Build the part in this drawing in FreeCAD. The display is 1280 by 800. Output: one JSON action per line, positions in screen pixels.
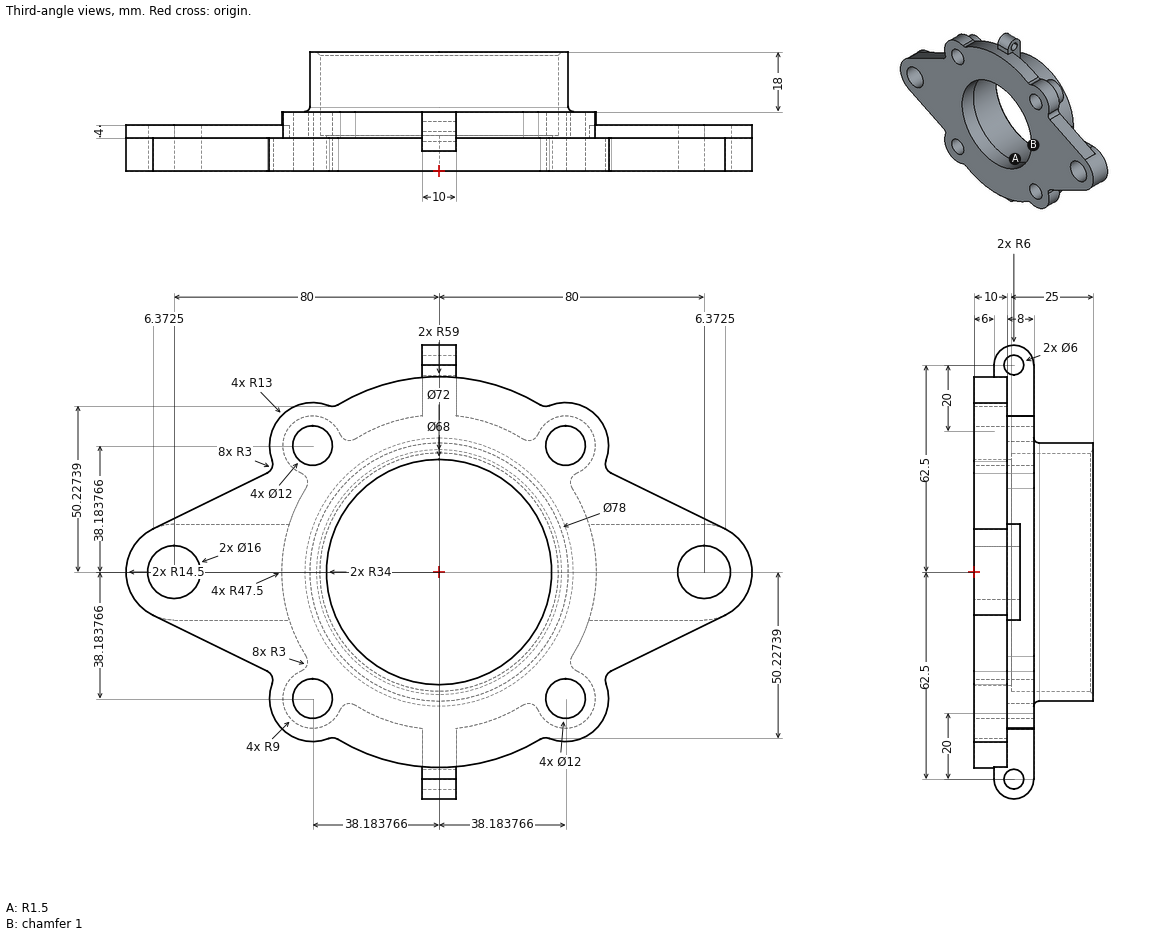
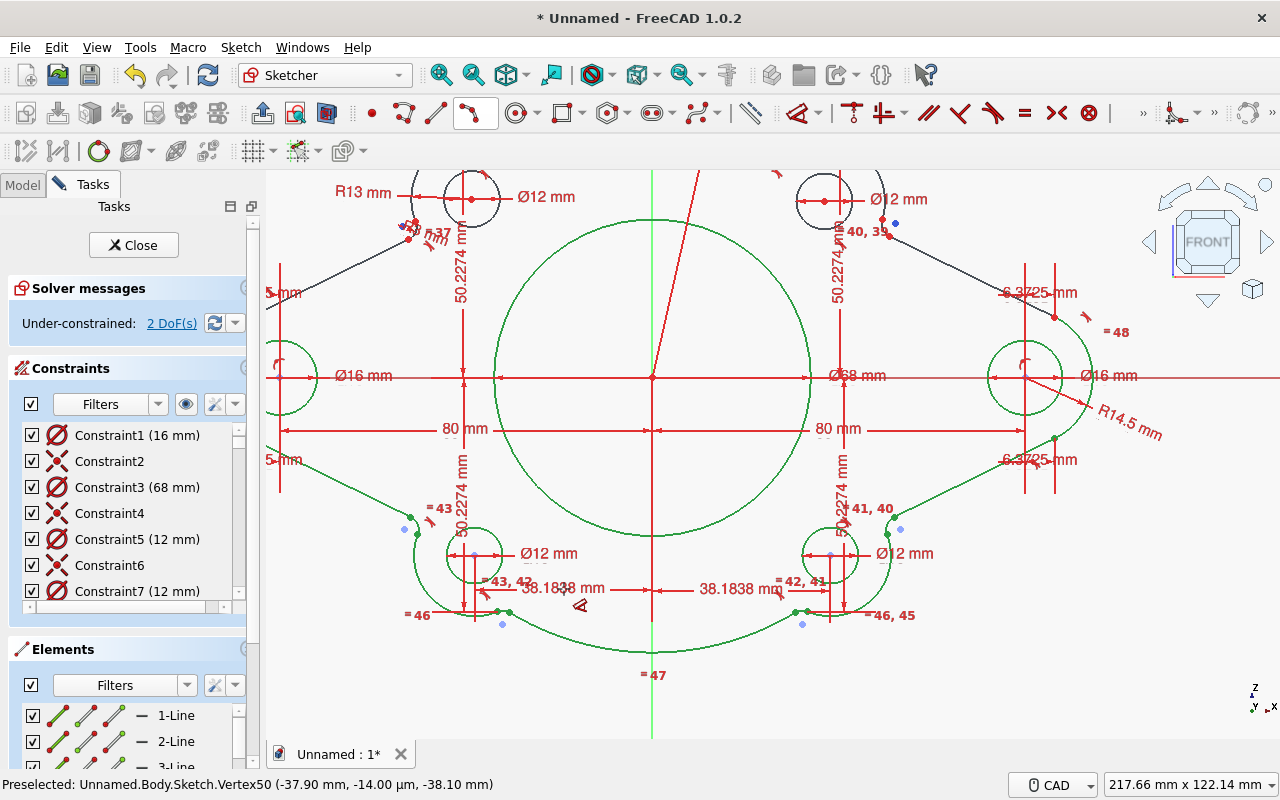
{"action": "left_click", "coordinate": [824, 201]}
{"action": "left_click", "coordinate": [738, 412]}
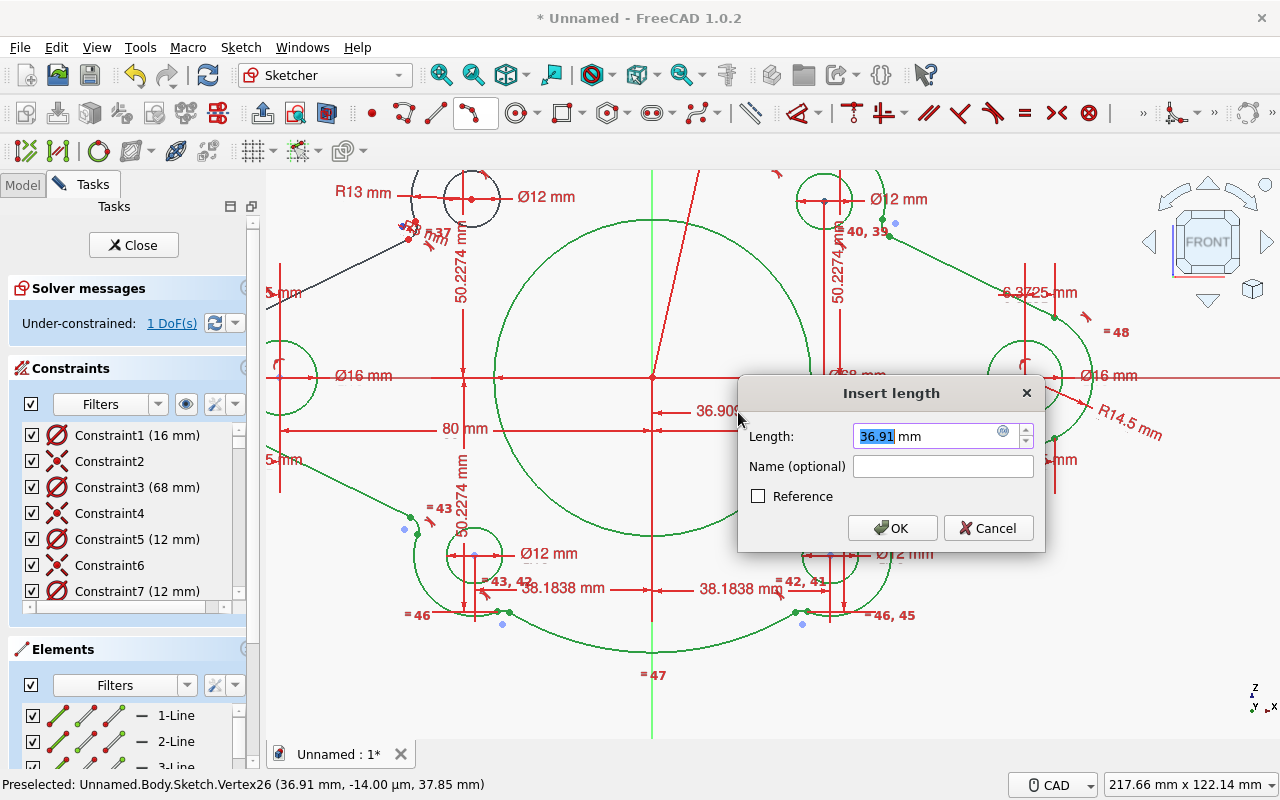
{"action": "type", "text": "38.183766"}
{"action": "key", "text": "Return"}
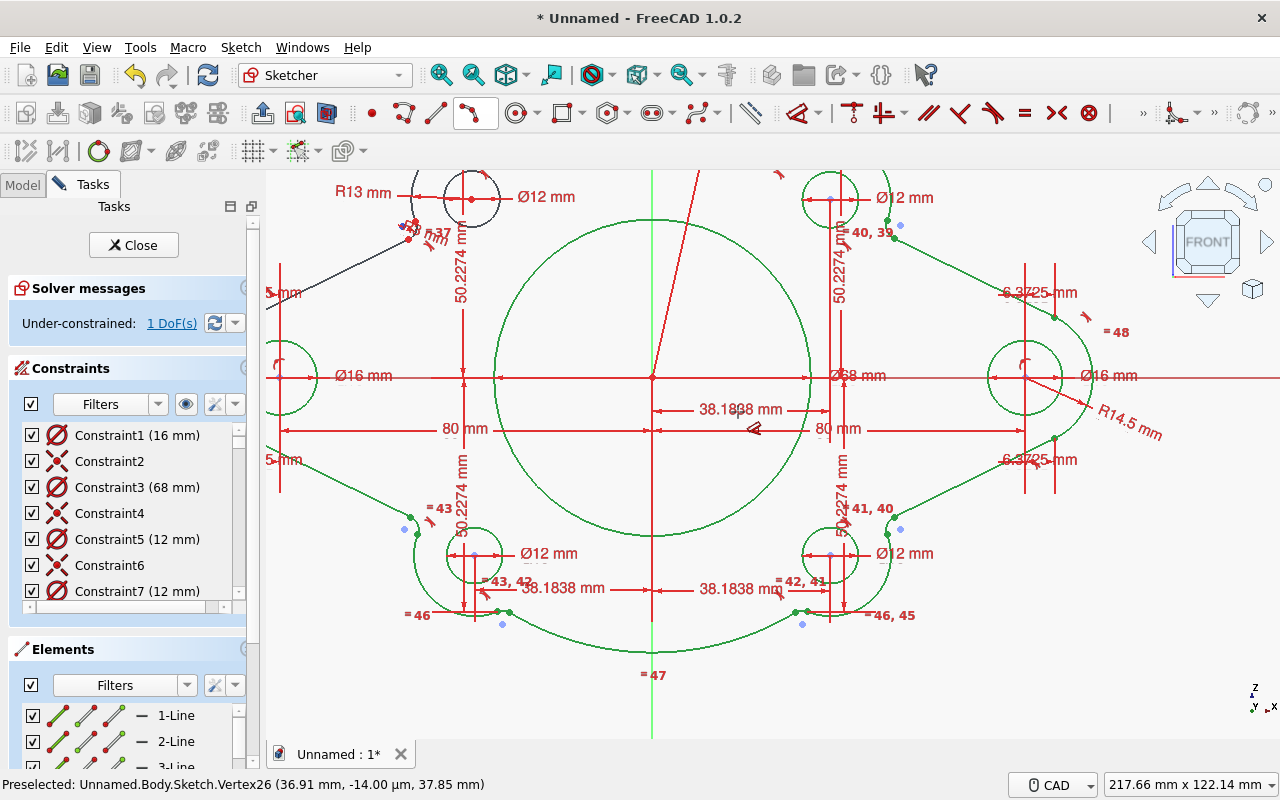
{"action": "left_click", "coordinate": [472, 199]}
{"action": "left_click", "coordinate": [562, 412]}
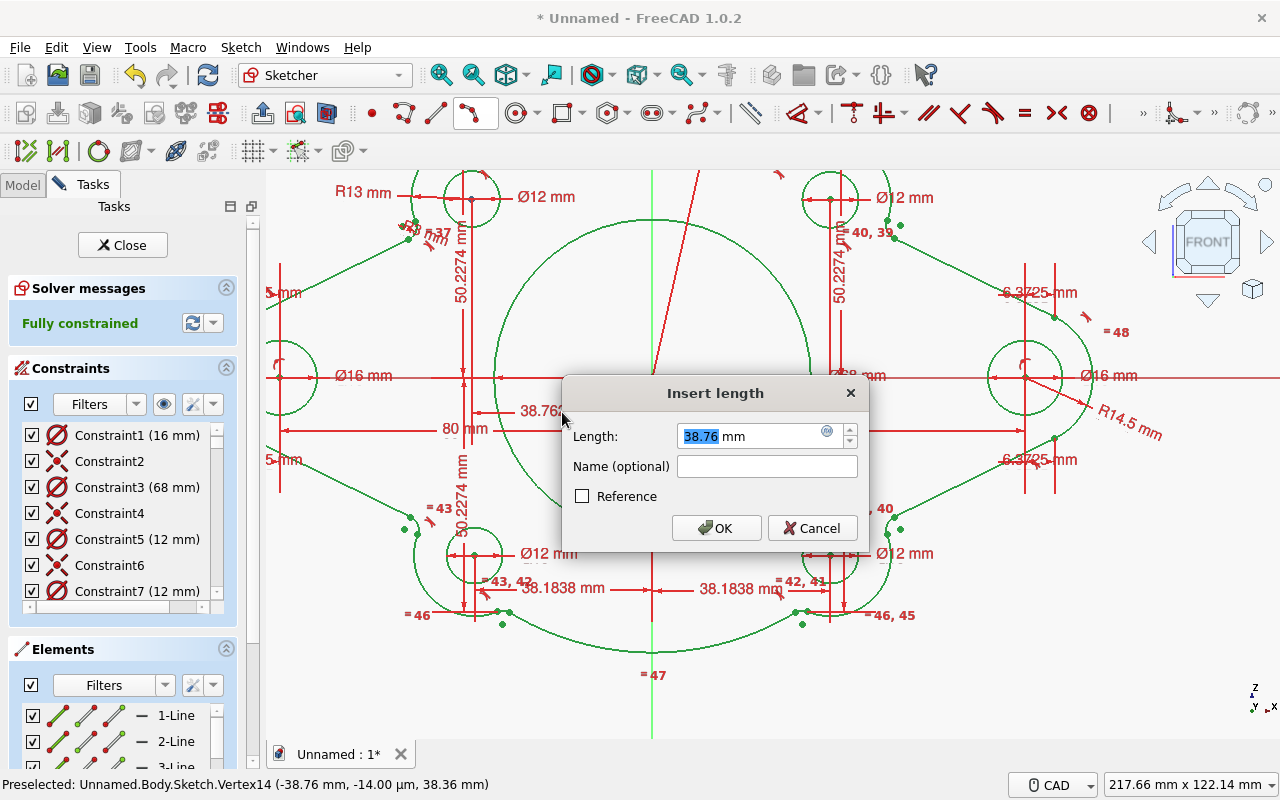
{"action": "type", "text": "38.183766"}
{"action": "key", "text": "Return"}
{"action": "key", "text": "Escape"}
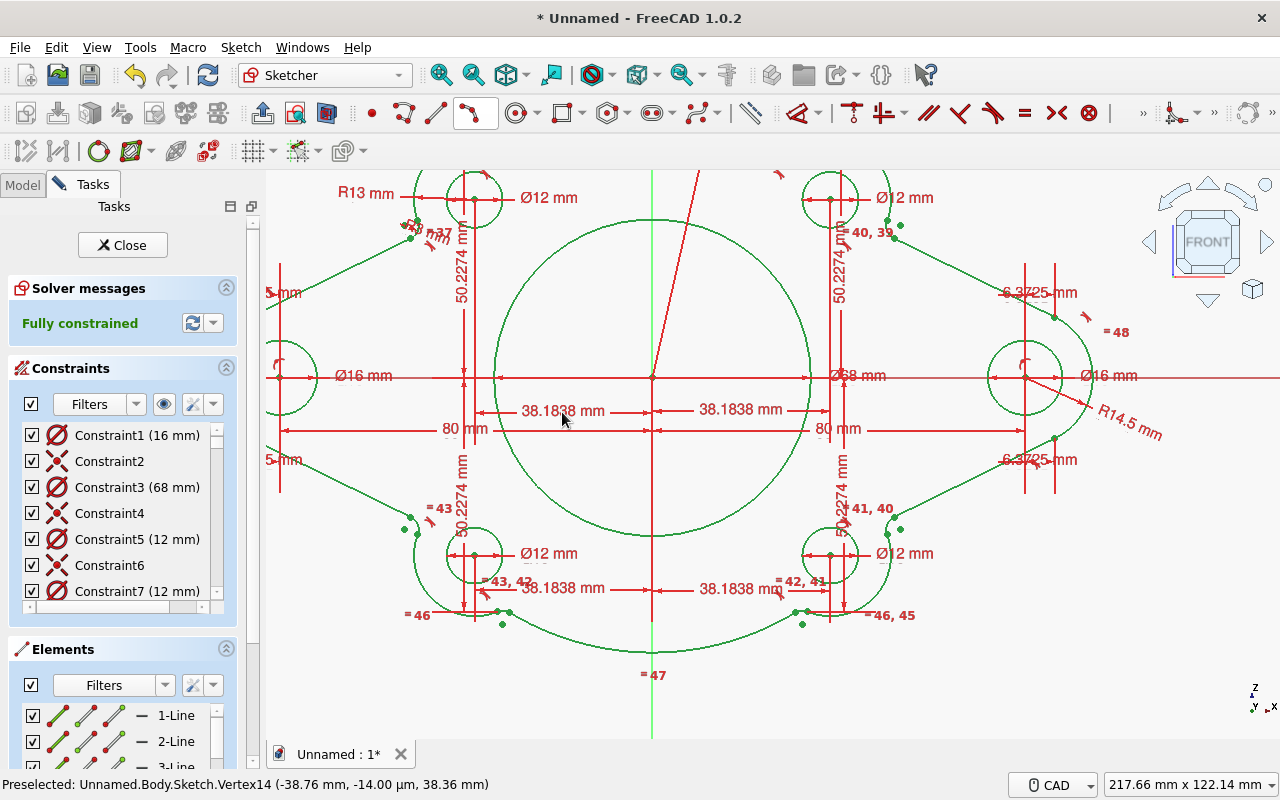
{"action": "left_click", "coordinate": [123, 245]}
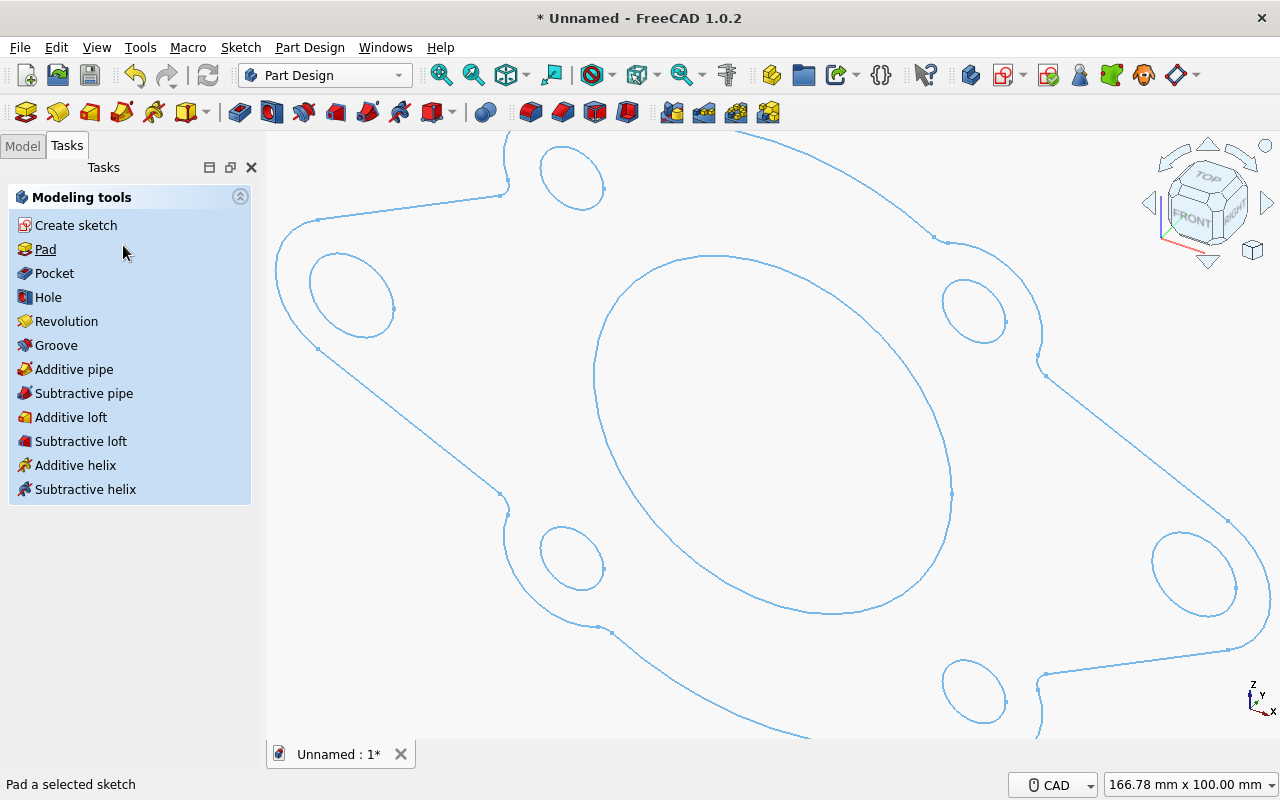
{"action": "left_click", "coordinate": [26, 112]}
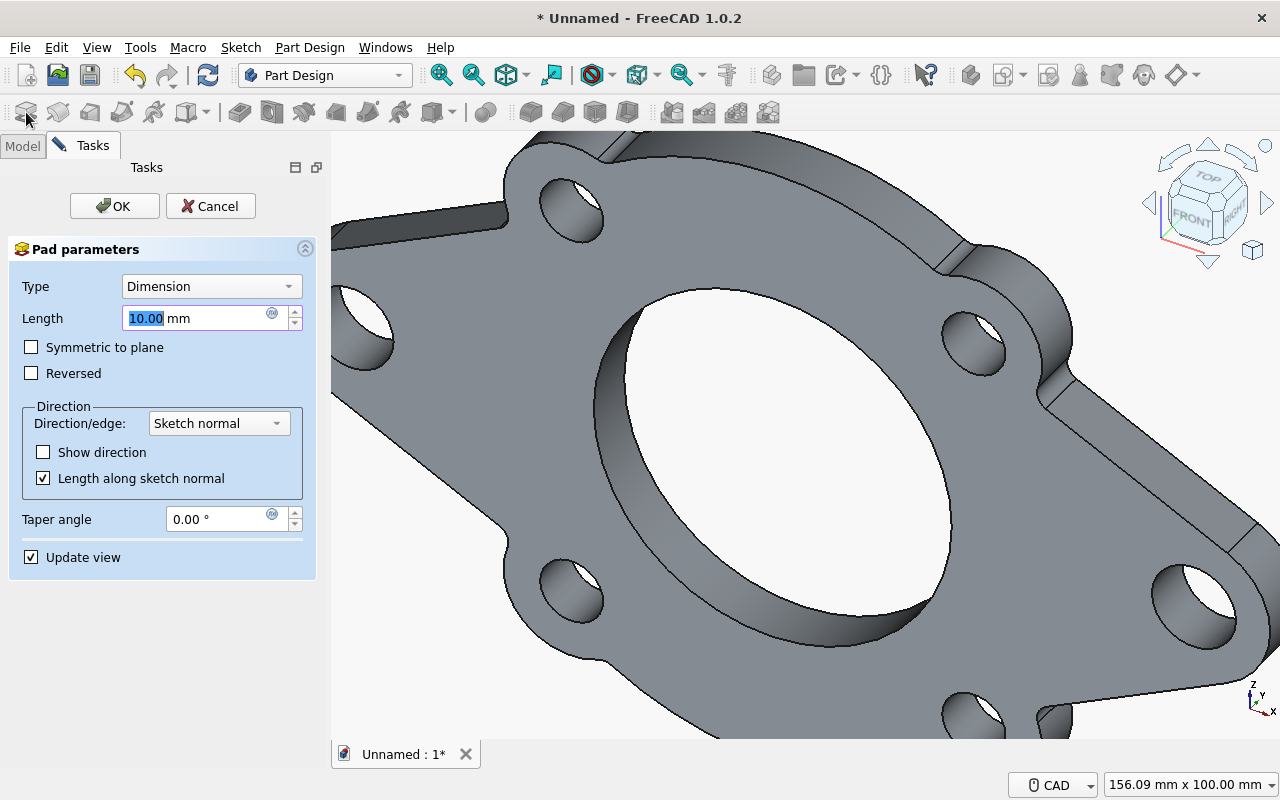
{"action": "type", "text": "10"}
{"action": "key", "text": "Tab"}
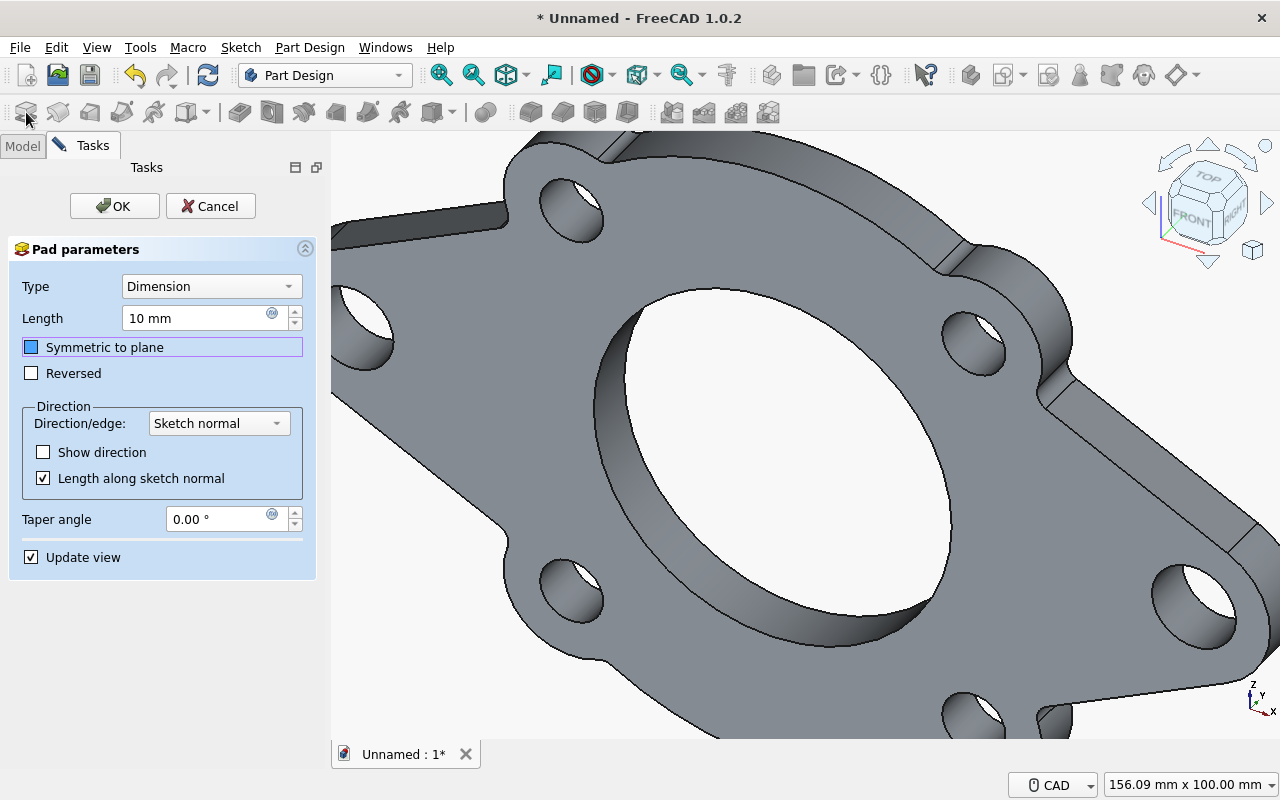
{"action": "left_click", "coordinate": [30, 373]}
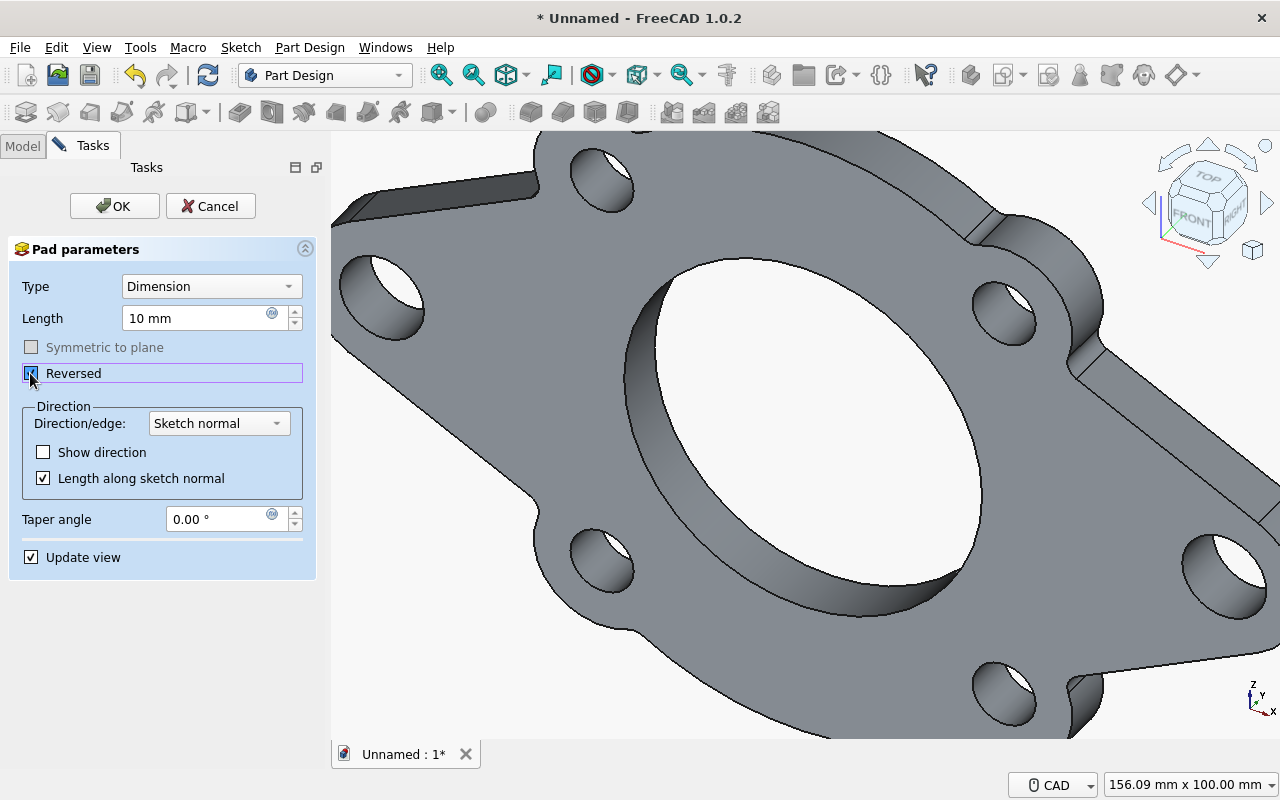
{"action": "left_click", "coordinate": [115, 206]}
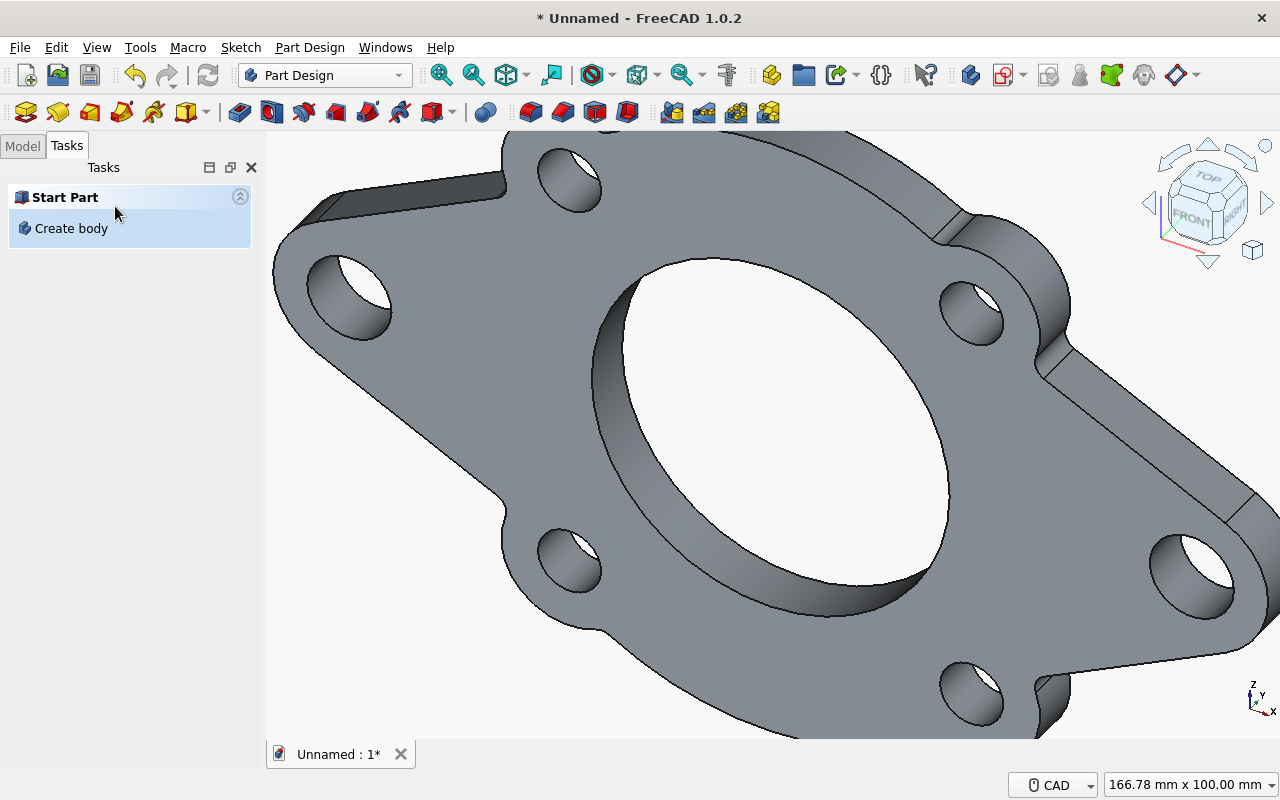
{"action": "left_click", "coordinate": [442, 76]}